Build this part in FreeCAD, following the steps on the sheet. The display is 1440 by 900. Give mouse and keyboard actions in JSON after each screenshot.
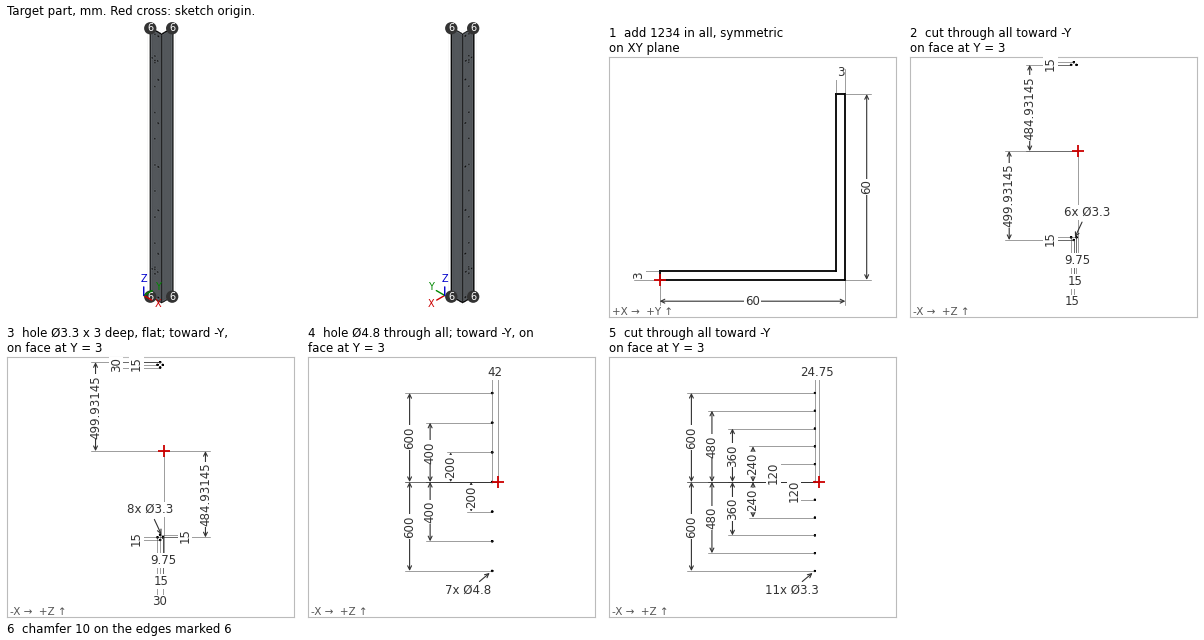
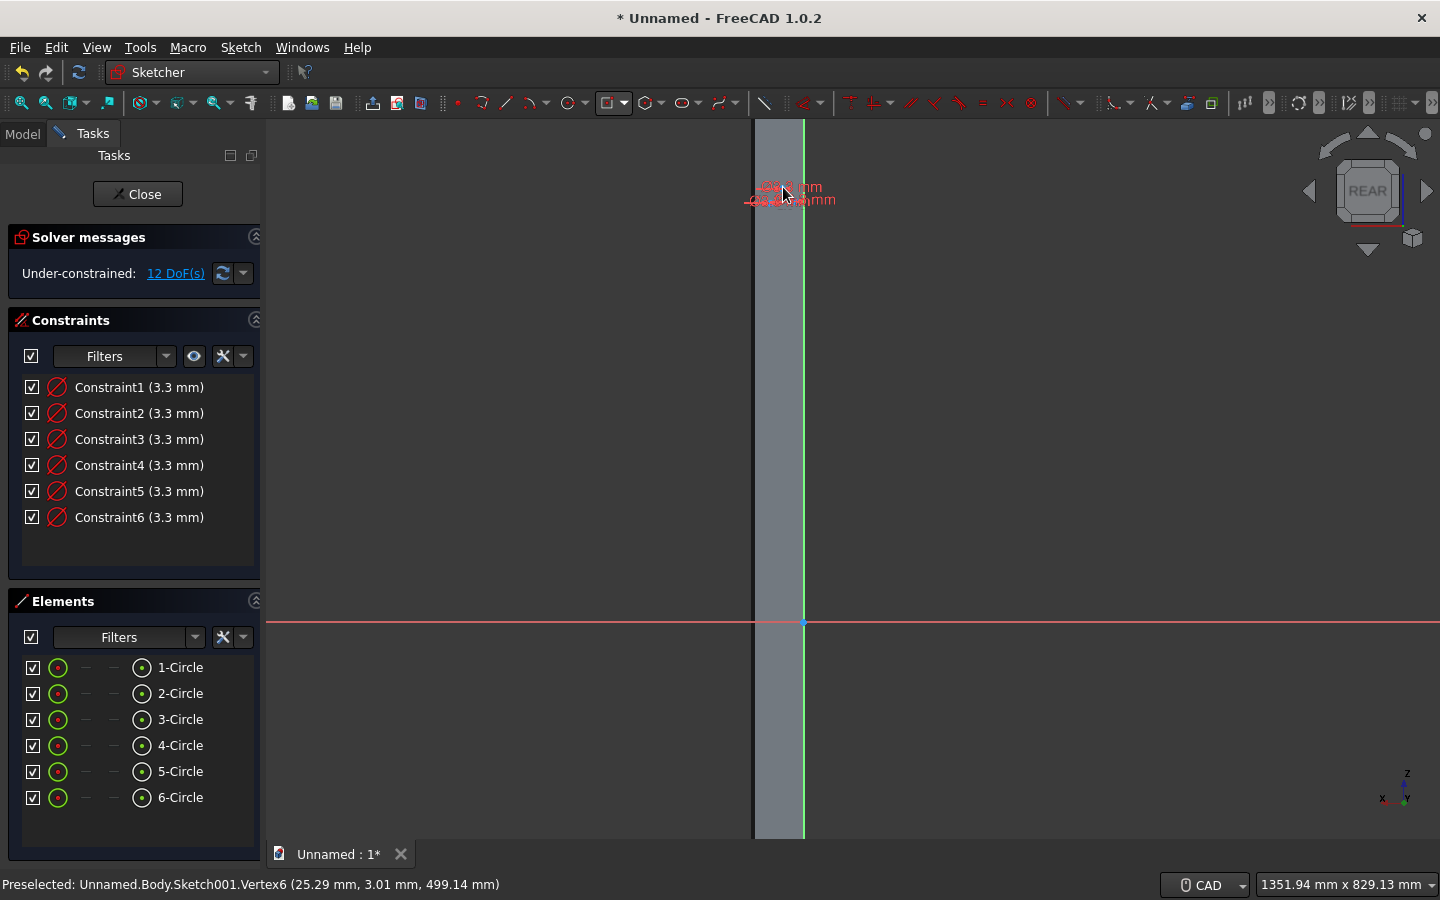
{"action": "scroll", "coordinate": [783, 305], "scroll_direction": "down", "scroll_amount": 3}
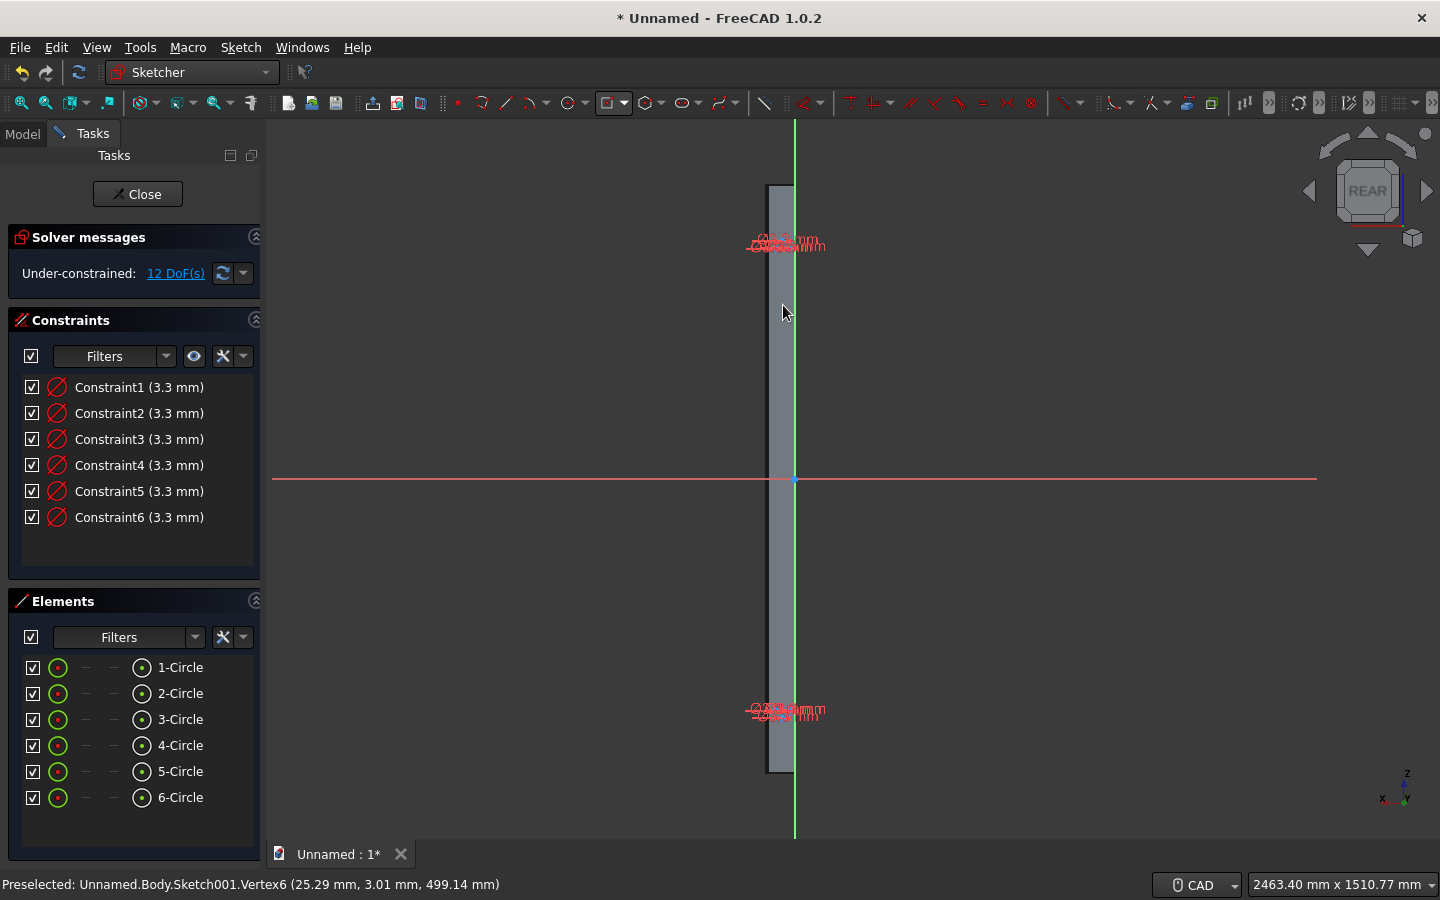
{"action": "left_click", "coordinate": [790, 711]}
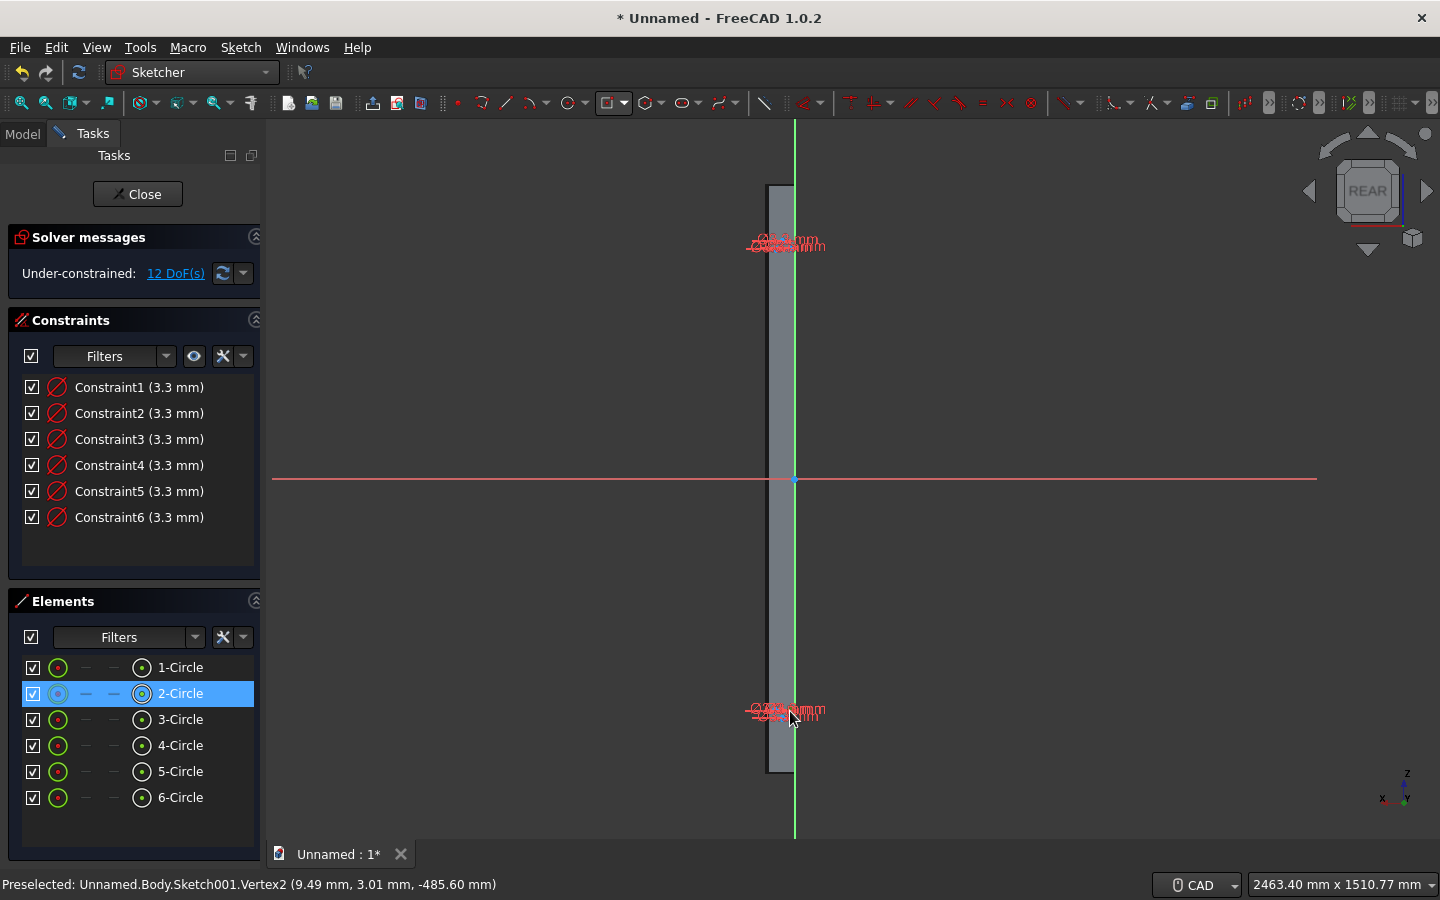
{"action": "left_click", "coordinate": [776, 711]}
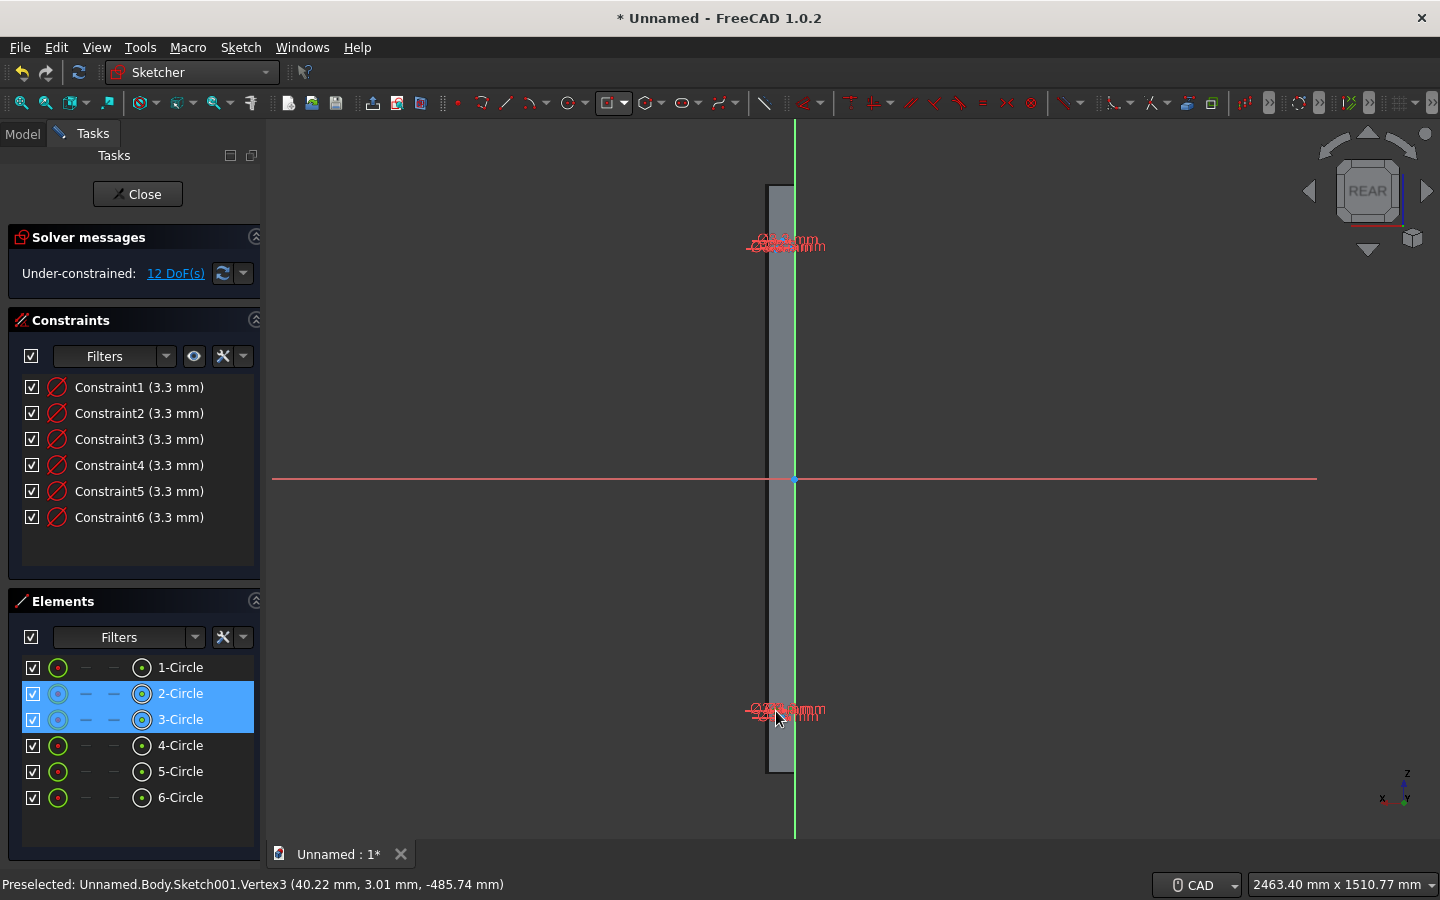
{"action": "left_click", "coordinate": [892, 104]}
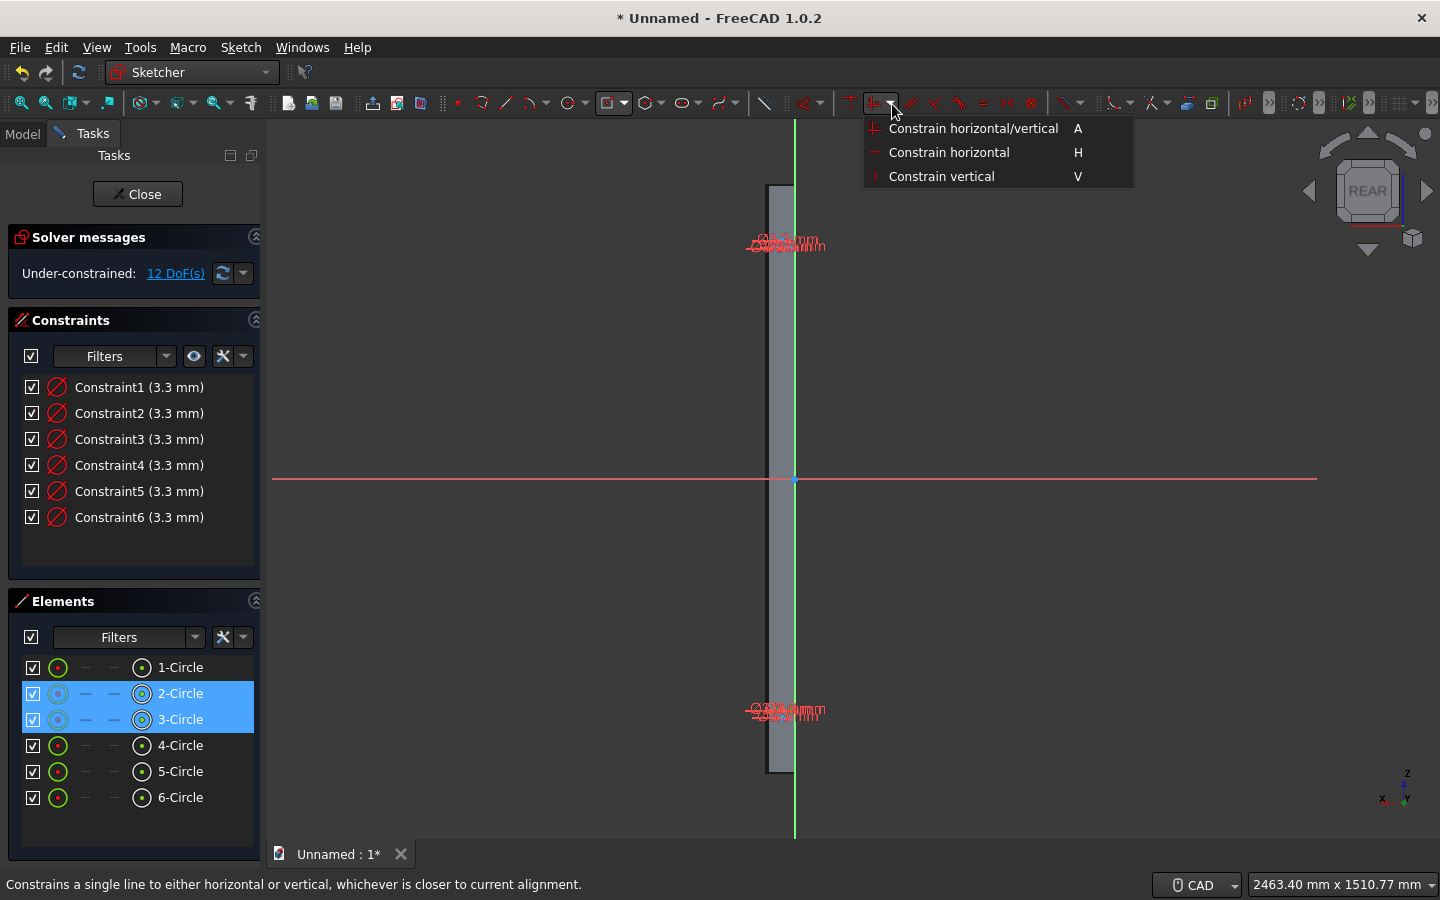
{"action": "left_click", "coordinate": [999, 152]}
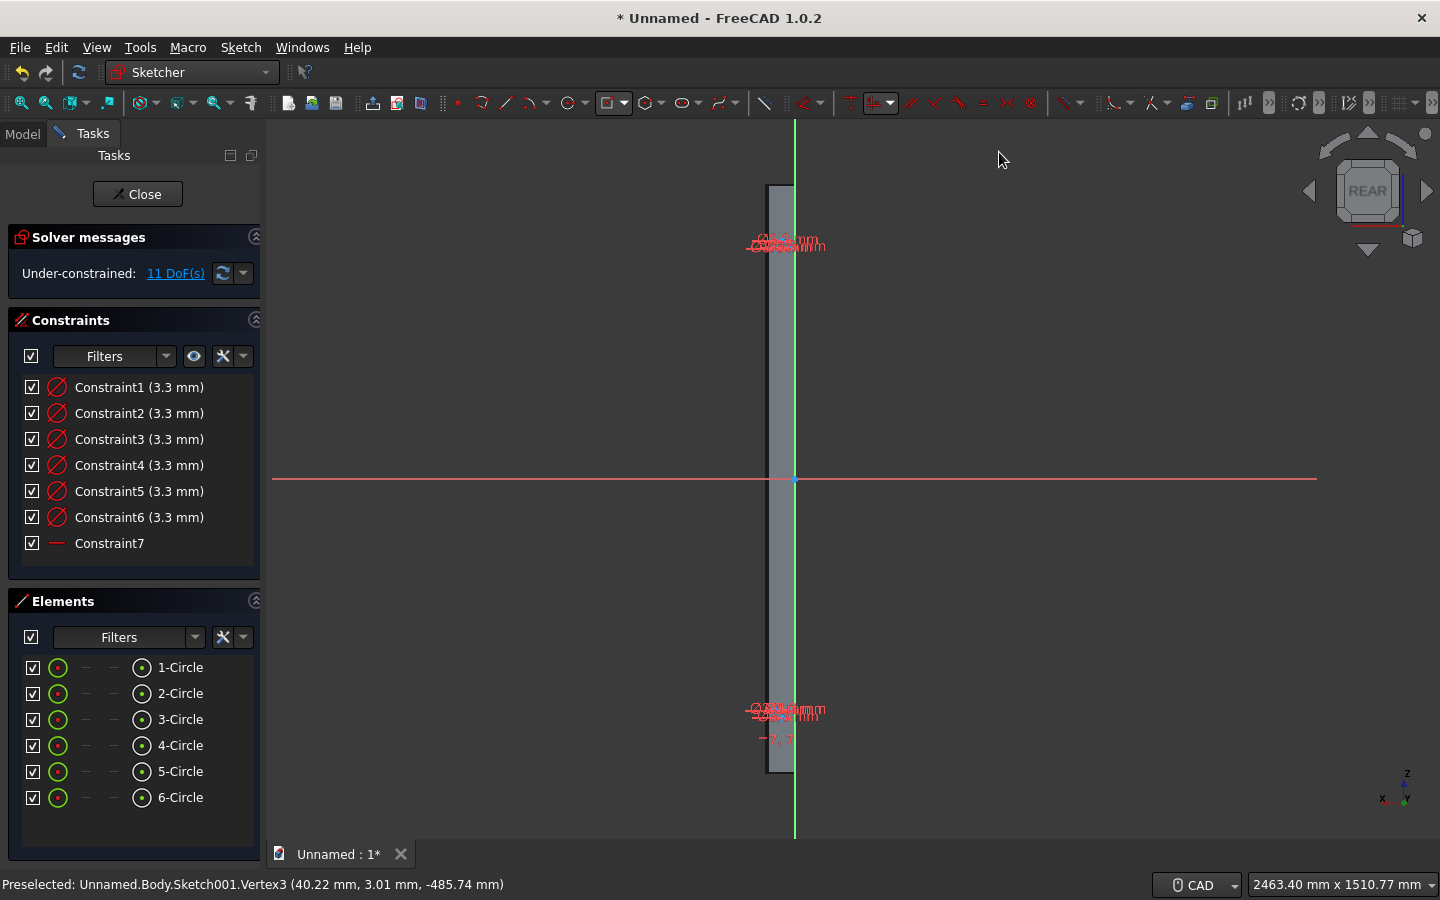
{"action": "left_click", "coordinate": [776, 711]}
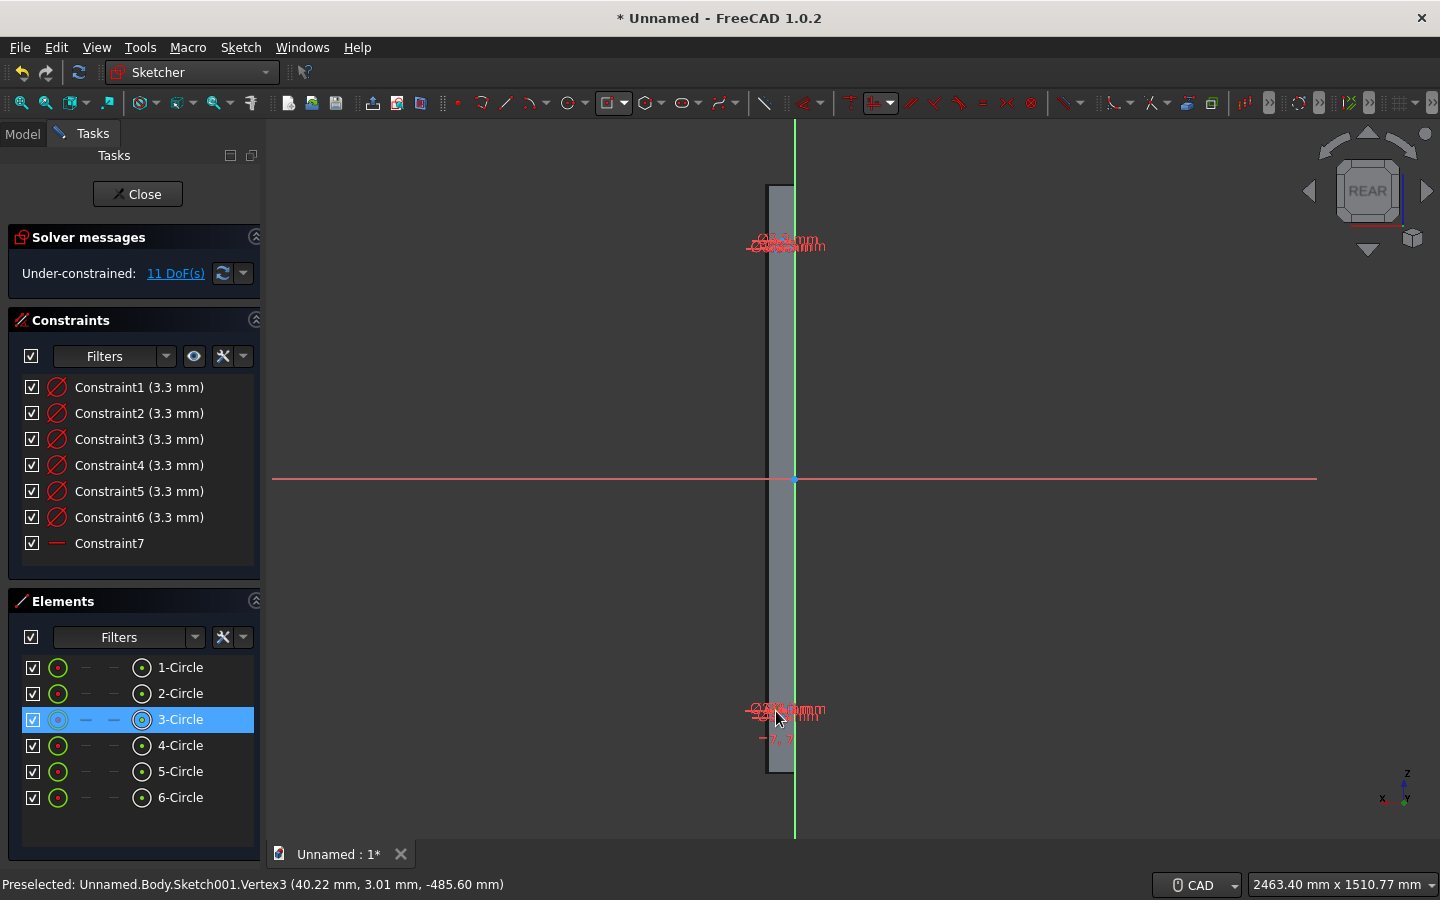
{"action": "left_click", "coordinate": [776, 249]}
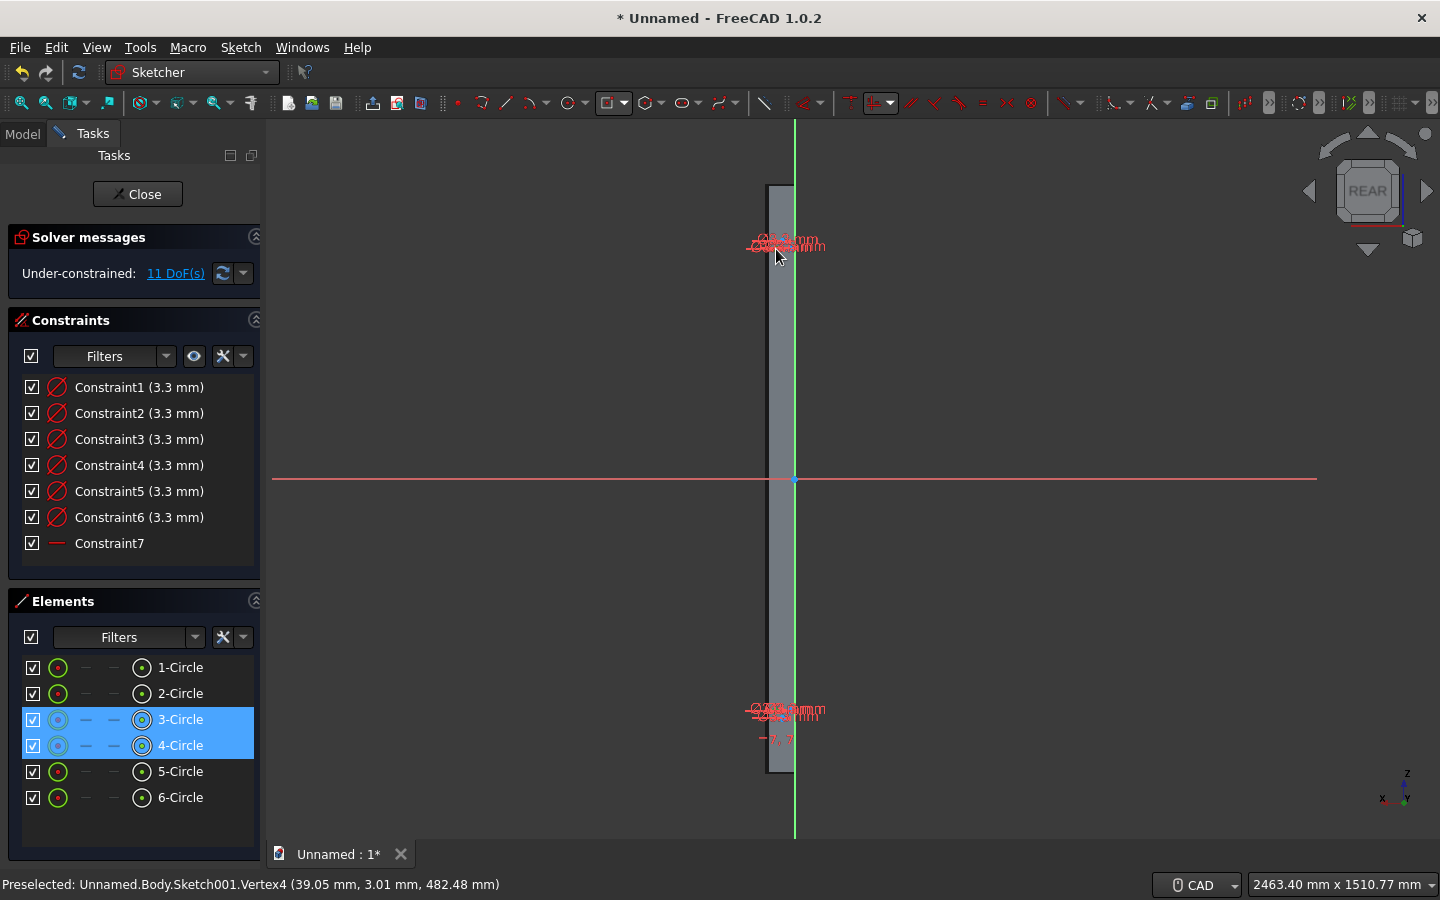
{"action": "left_click", "coordinate": [892, 104]}